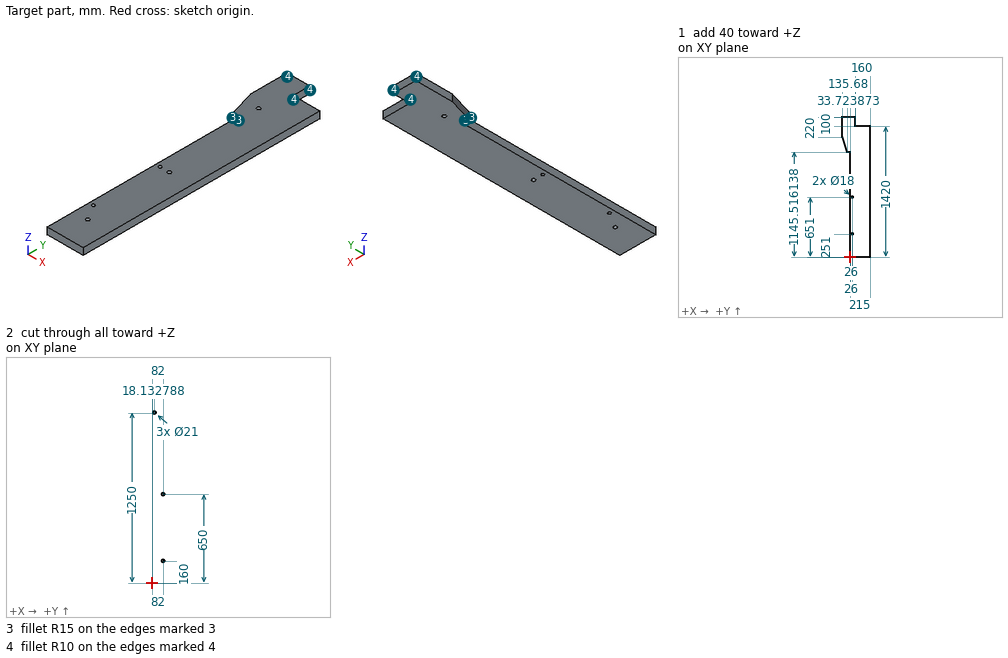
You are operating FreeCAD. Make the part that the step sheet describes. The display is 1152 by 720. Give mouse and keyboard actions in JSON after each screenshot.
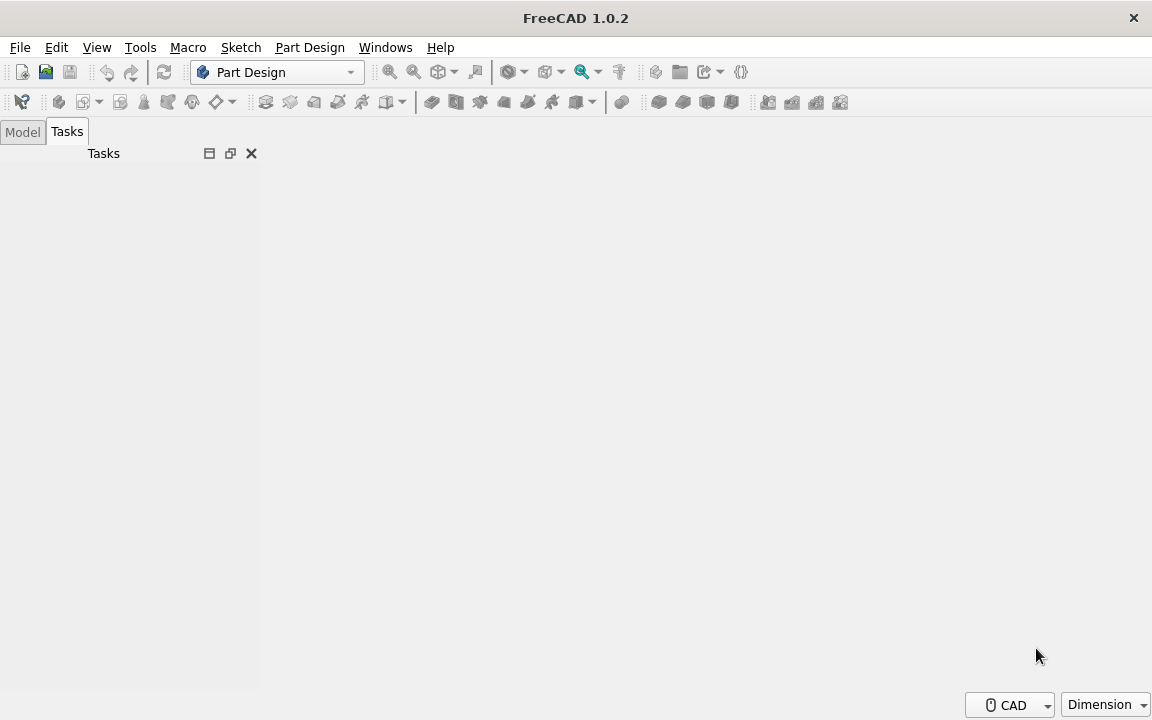
{"action": "key", "text": "ctrl+n"}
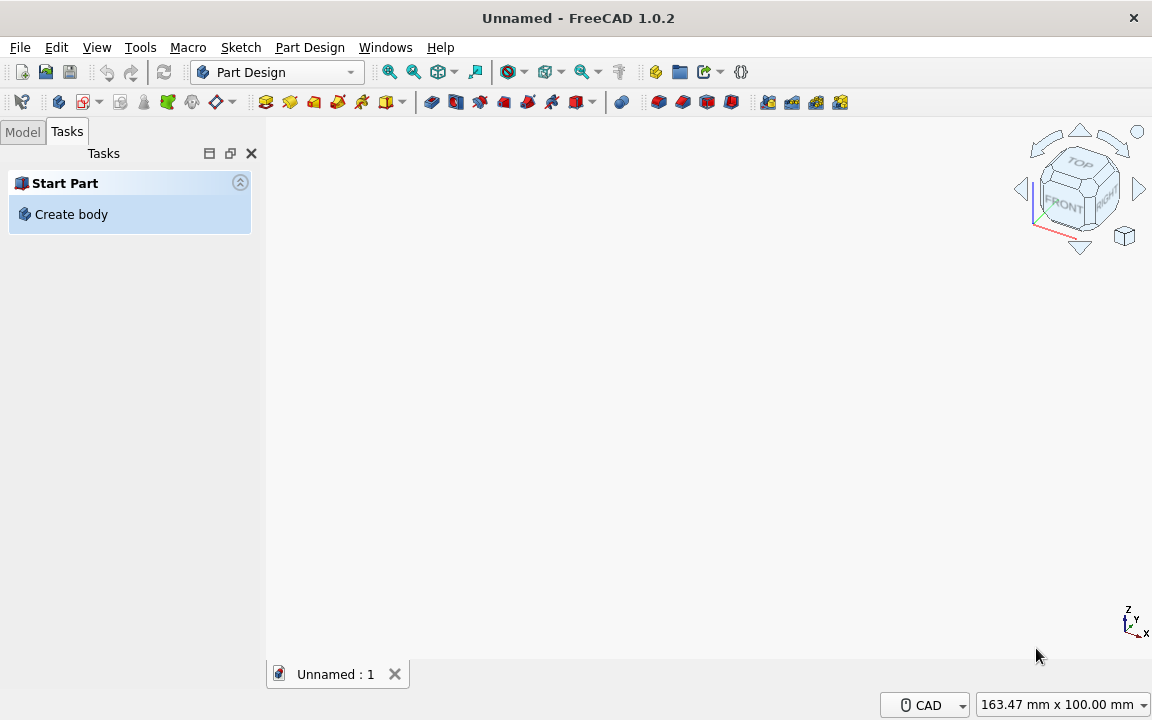
{"action": "left_click", "coordinate": [84, 102]}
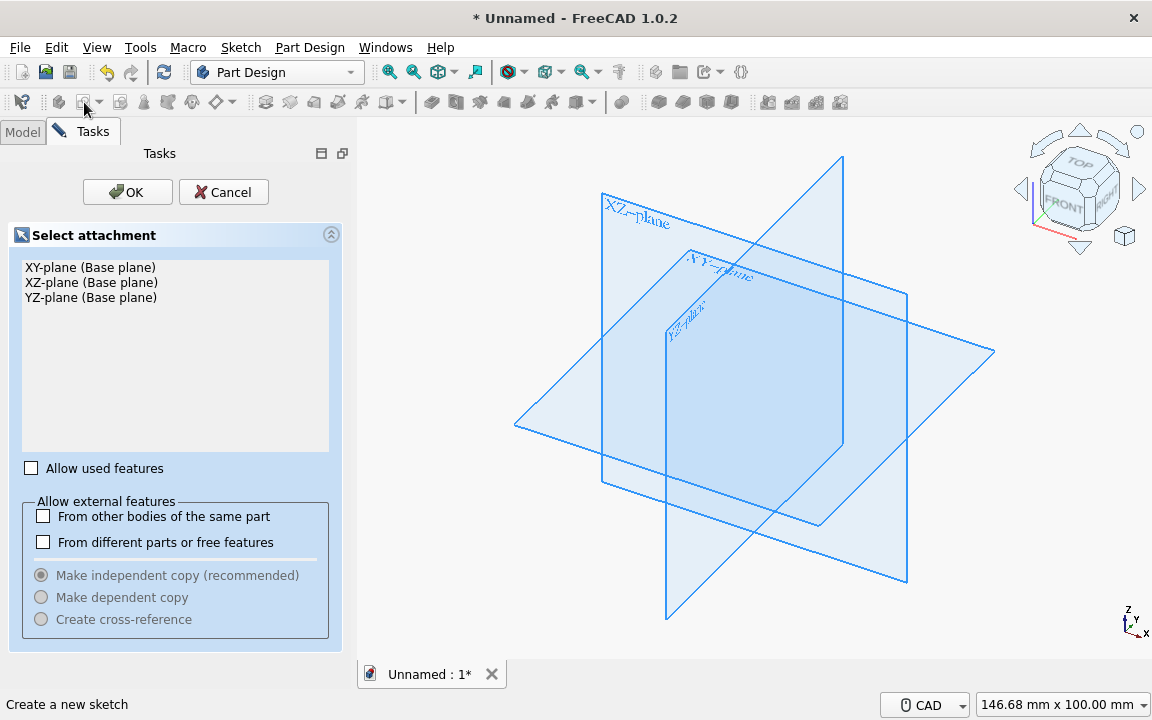
{"action": "left_click", "coordinate": [82, 268]}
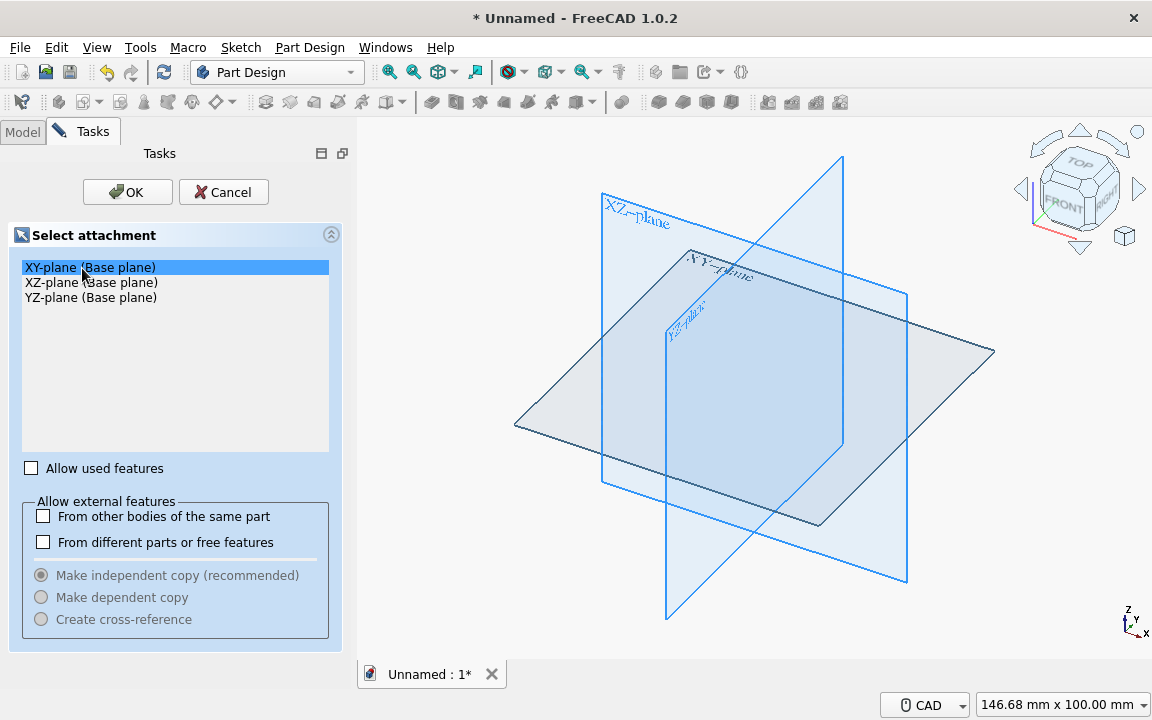
{"action": "left_click", "coordinate": [128, 192]}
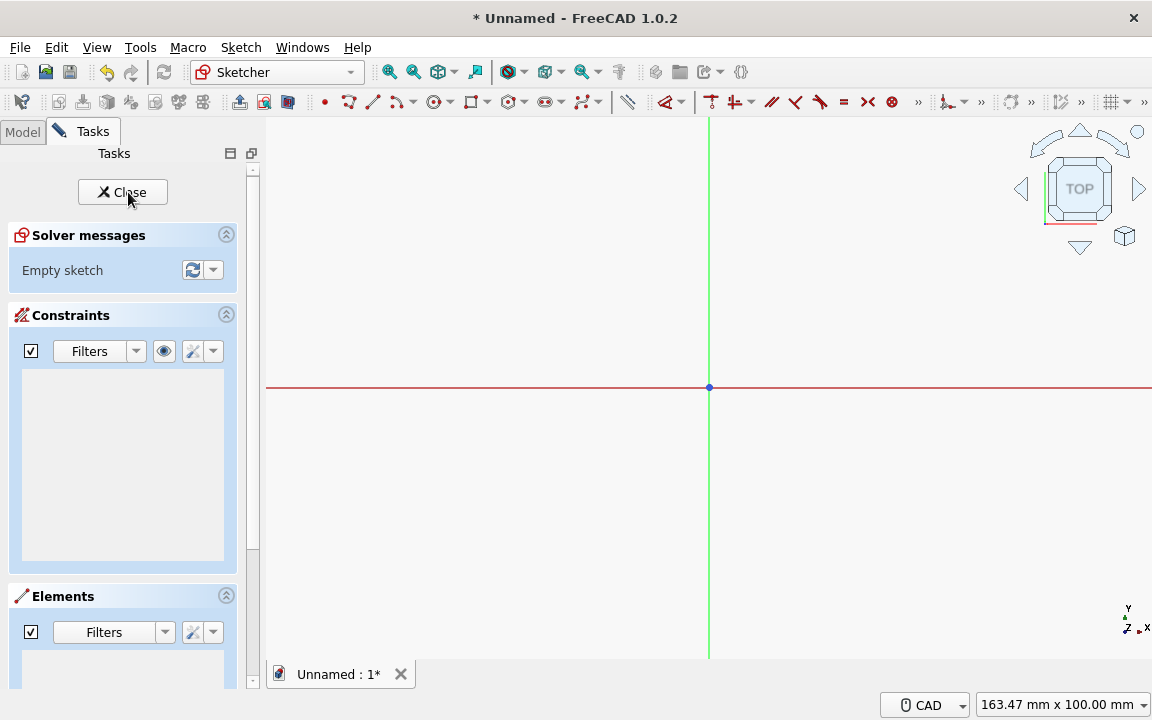
{"action": "scroll", "coordinate": [618, 604], "scroll_direction": "down", "scroll_amount": 15}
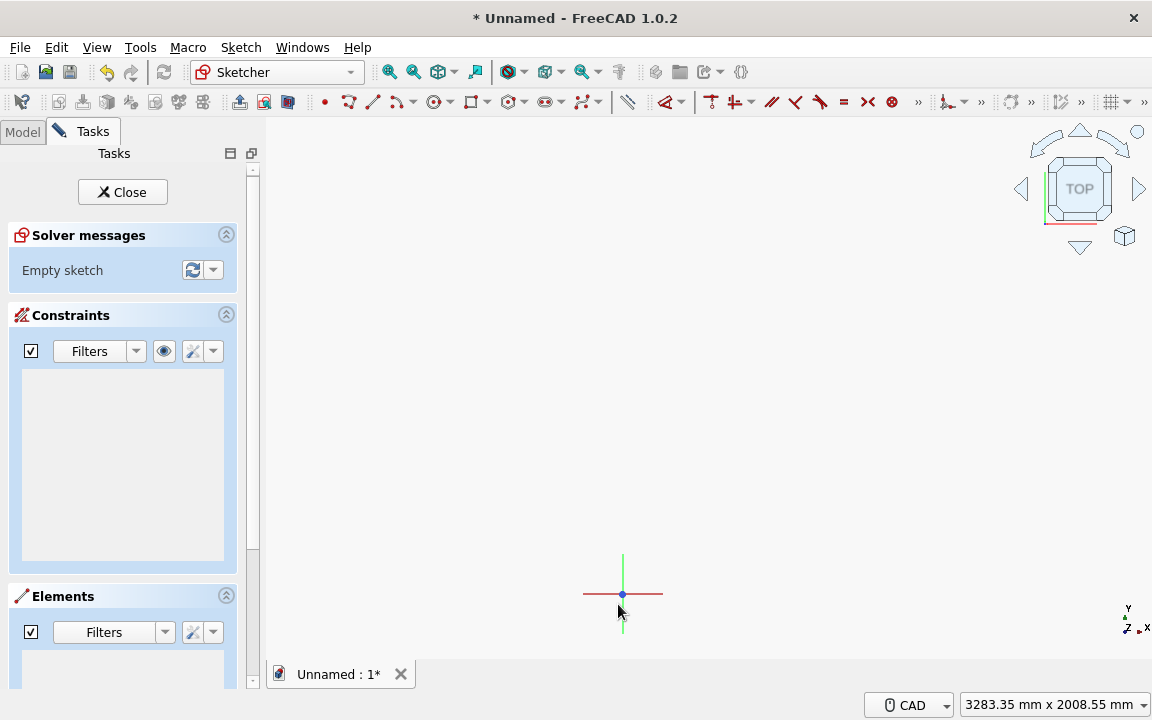
{"action": "key", "text": "g m"}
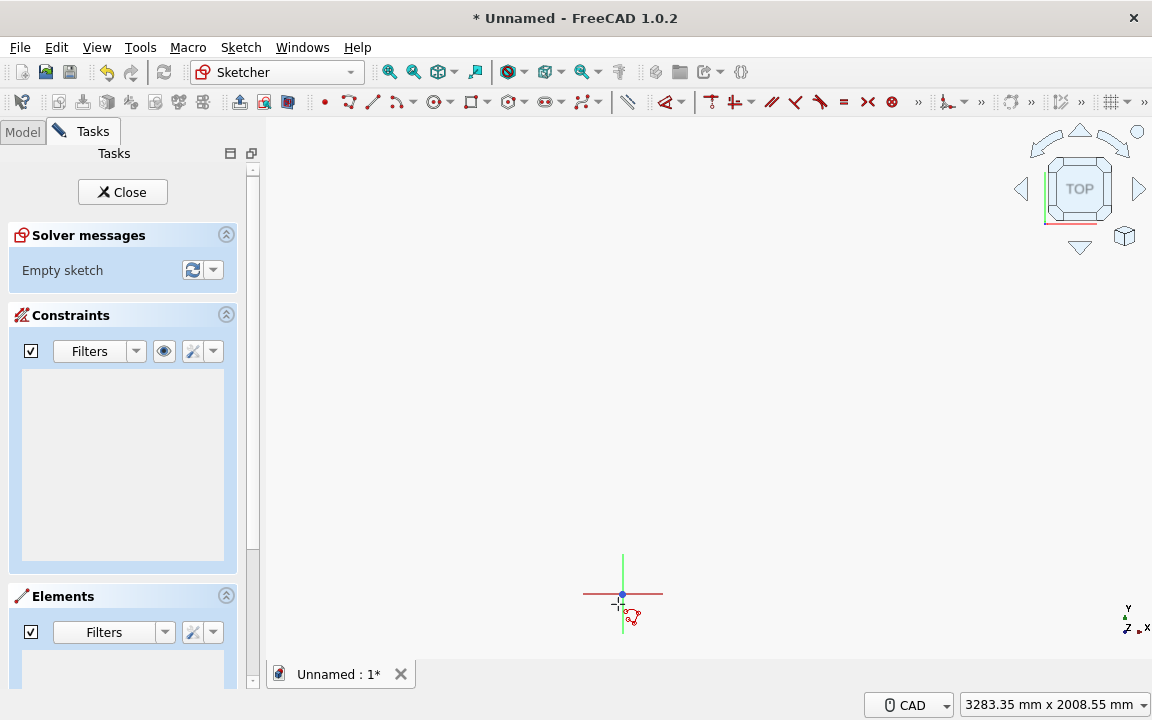
{"action": "left_click", "coordinate": [623, 594]}
{"action": "left_click", "coordinate": [681, 585]}
{"action": "left_click", "coordinate": [681, 211]}
{"action": "left_click", "coordinate": [638, 211]}
{"action": "left_click", "coordinate": [638, 184]}
{"action": "left_click", "coordinate": [601, 184]}
{"action": "left_click", "coordinate": [601, 243]}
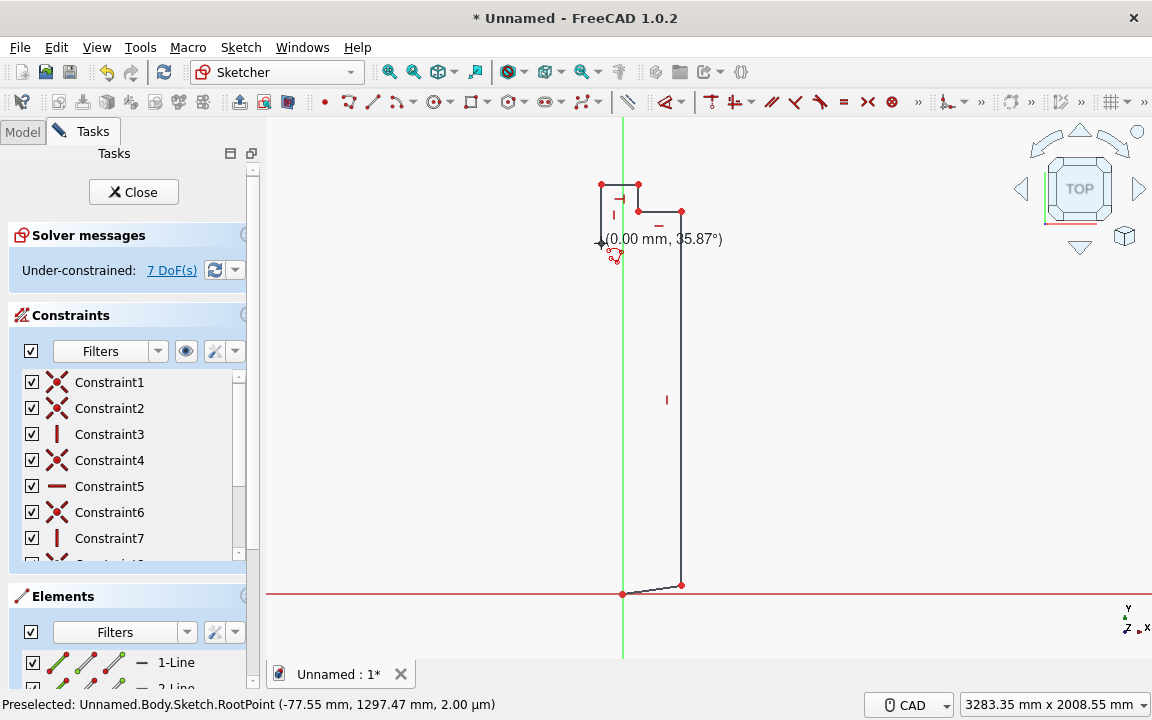
{"action": "scroll", "coordinate": [614, 285], "scroll_direction": "up", "scroll_amount": 3}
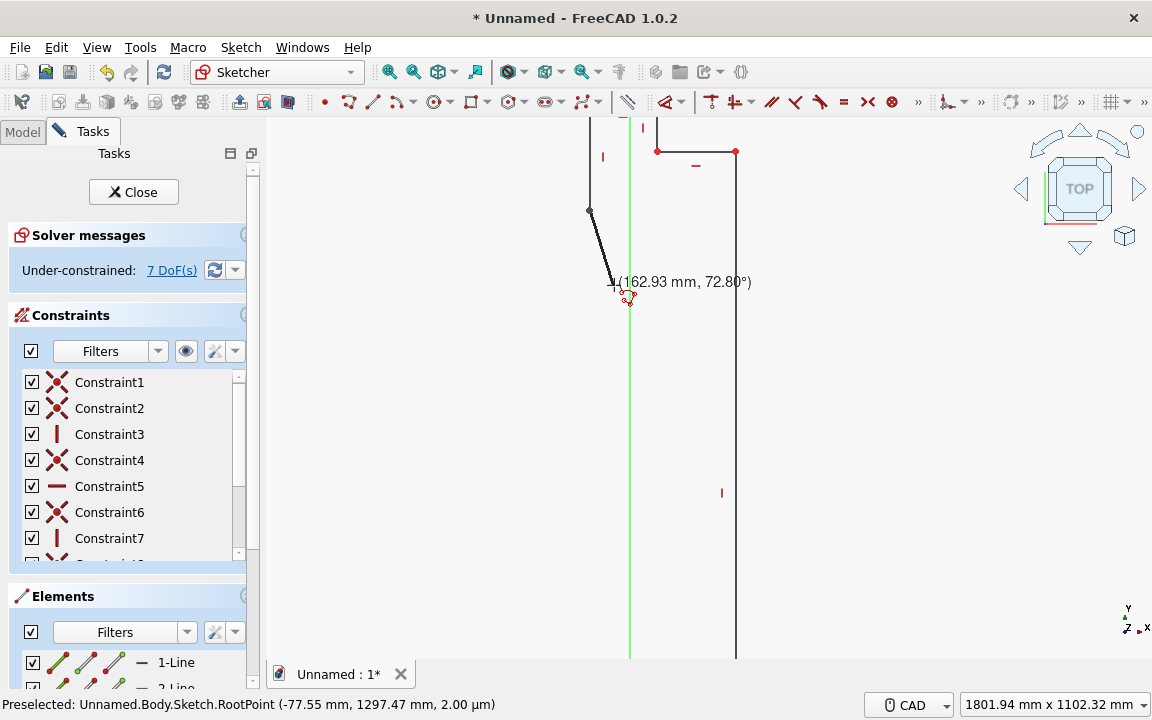
{"action": "left_click", "coordinate": [613, 285]}
{"action": "left_click", "coordinate": [639, 285]}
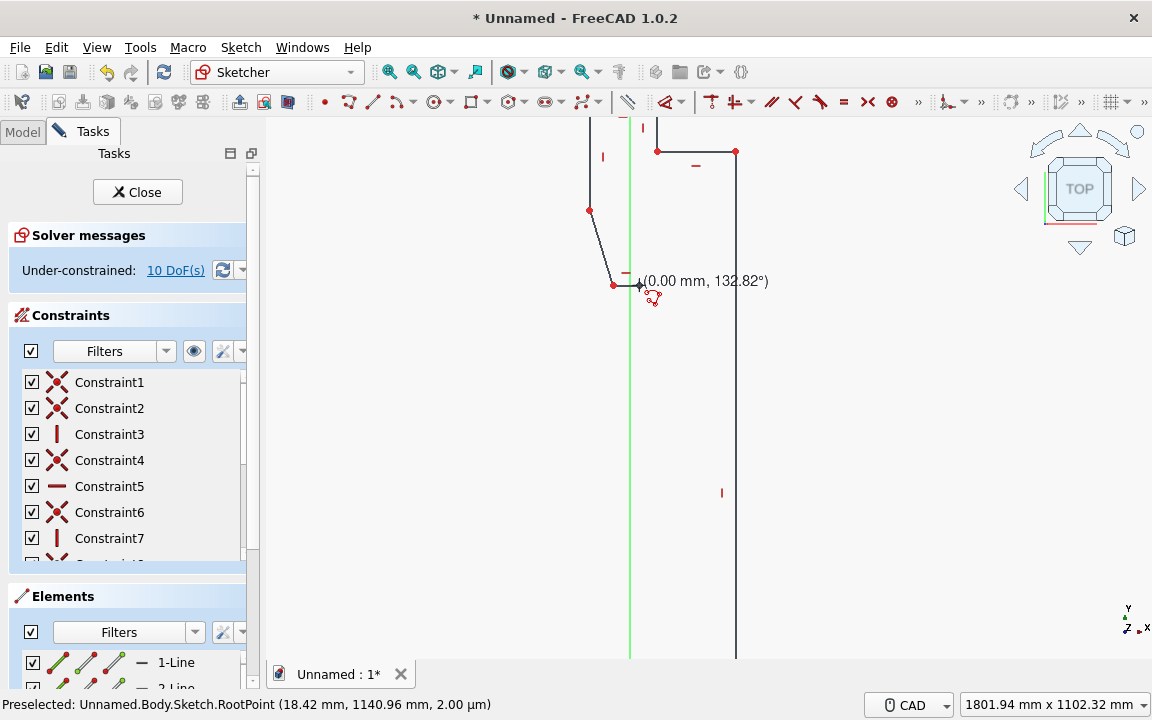
{"action": "scroll", "coordinate": [622, 318], "scroll_direction": "down", "scroll_amount": 4}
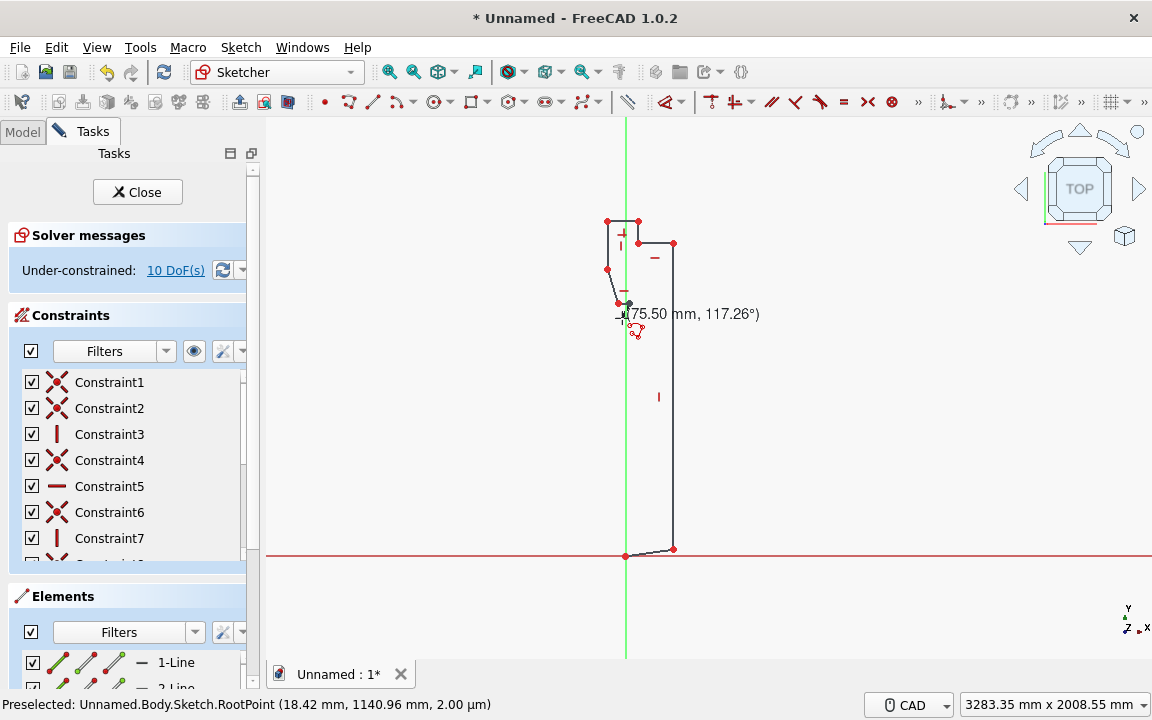
{"action": "left_click", "coordinate": [626, 556]}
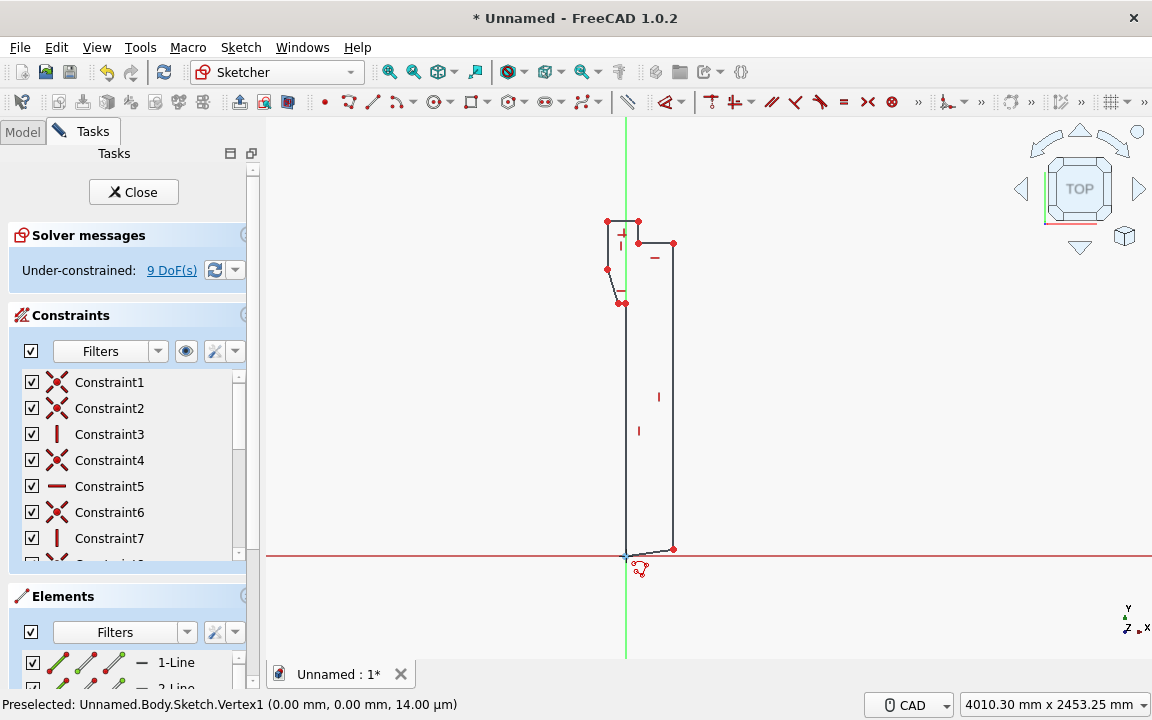
{"action": "key", "text": "g c"}